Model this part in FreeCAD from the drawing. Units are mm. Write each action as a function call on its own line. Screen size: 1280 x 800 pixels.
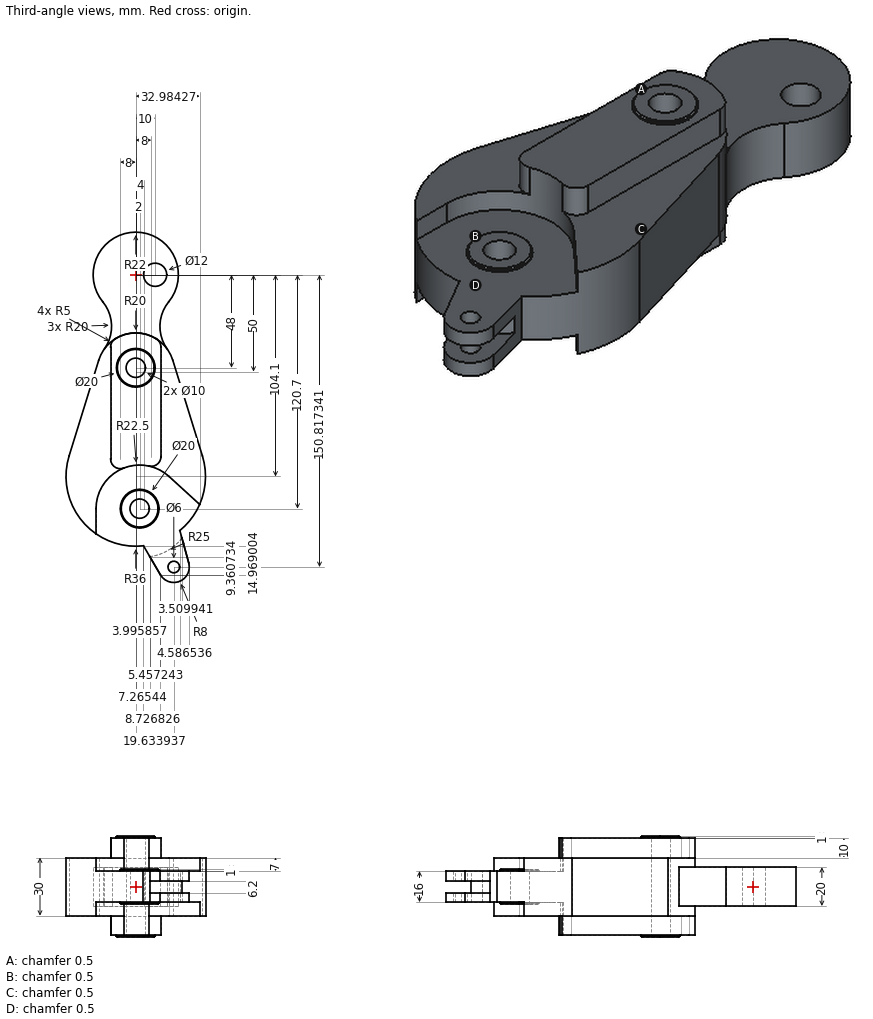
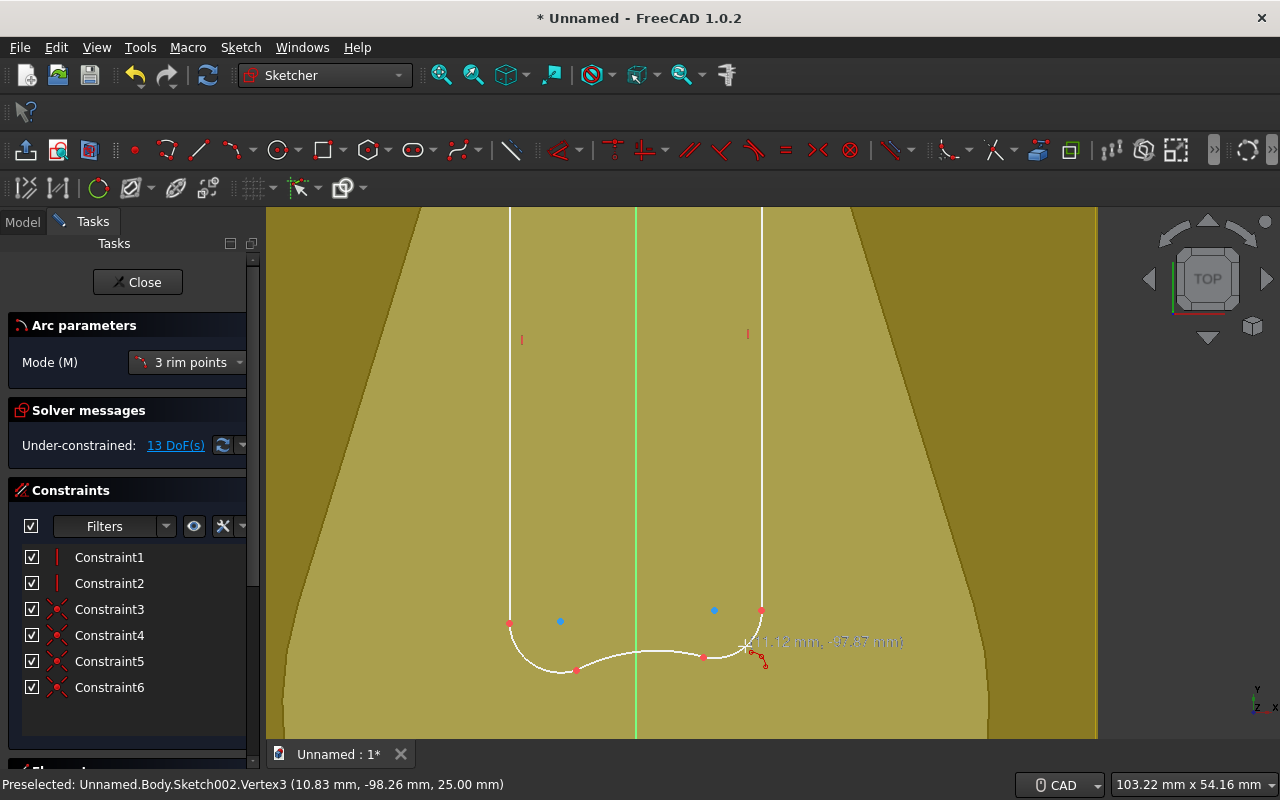
scroll(744, 646, down, 5)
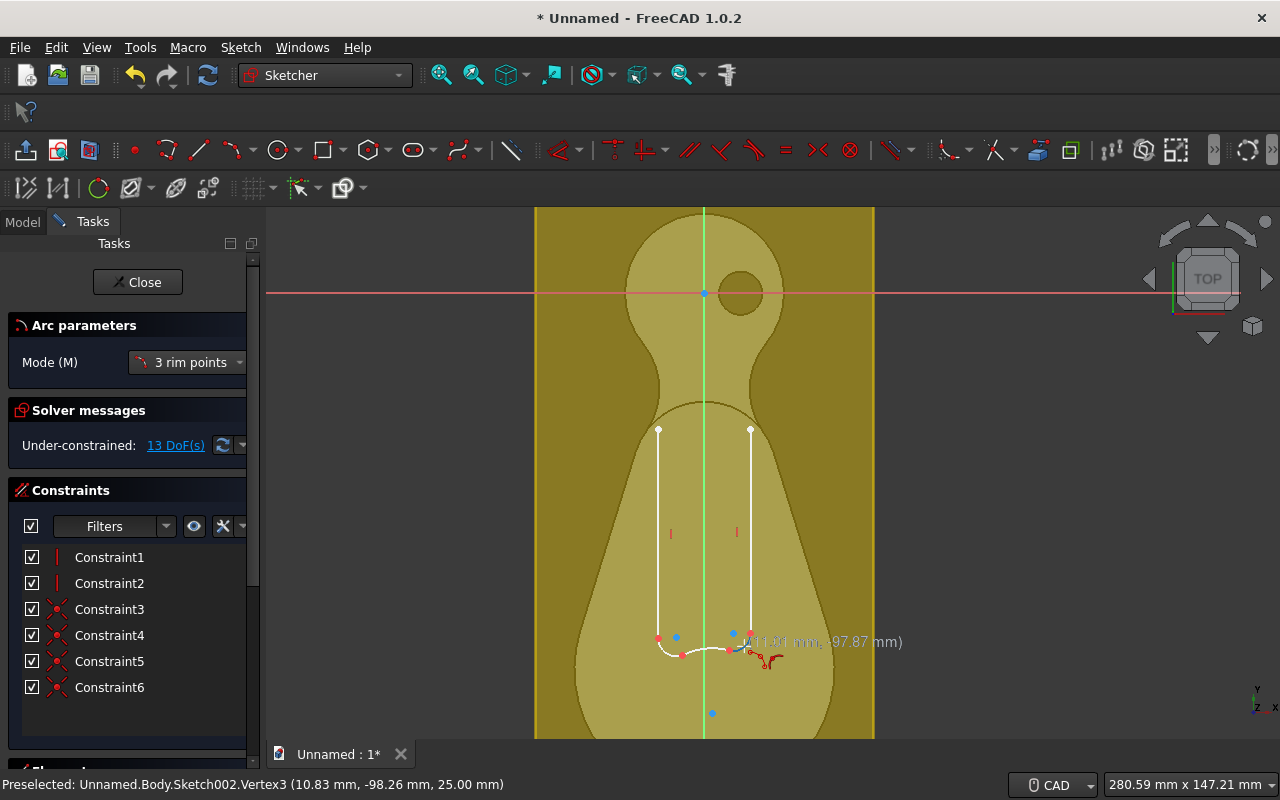
click(751, 430)
click(743, 413)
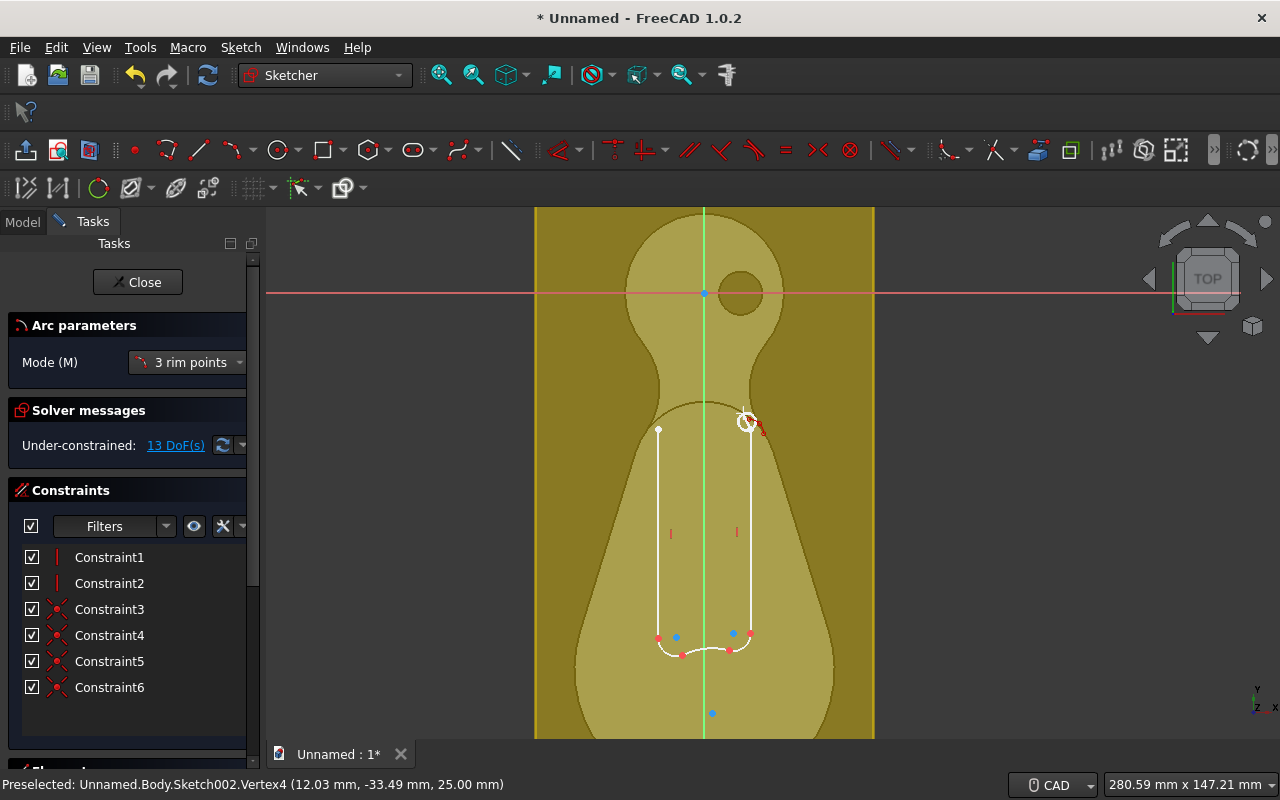
scroll(749, 419, up, 10)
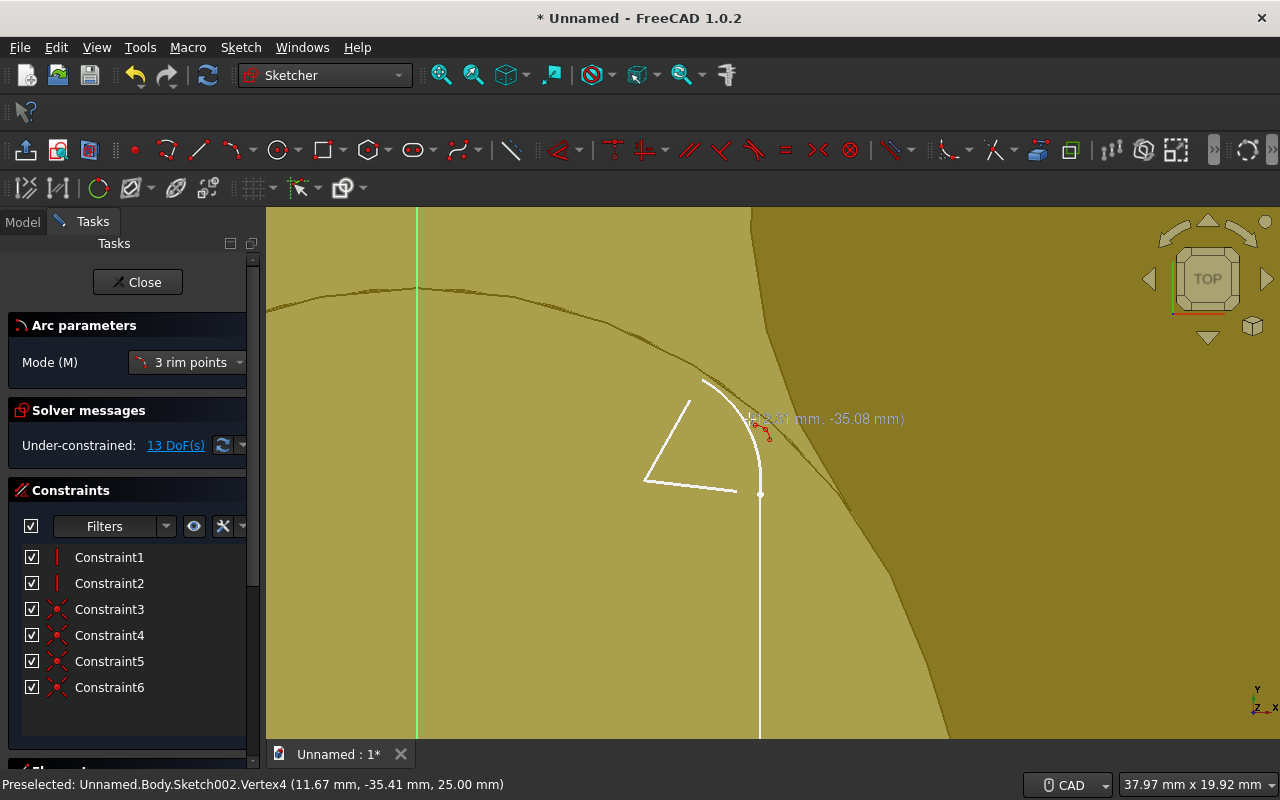
click(748, 419)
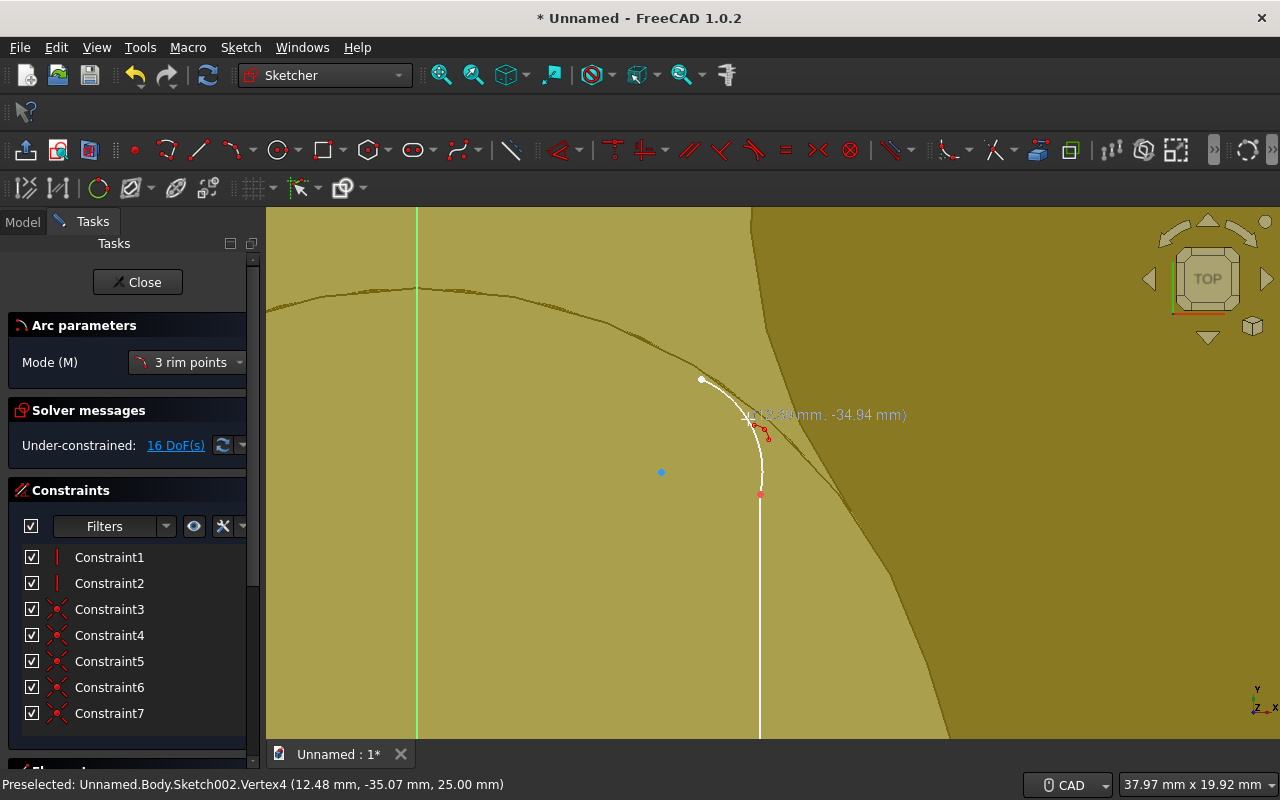
scroll(749, 419, down, 10)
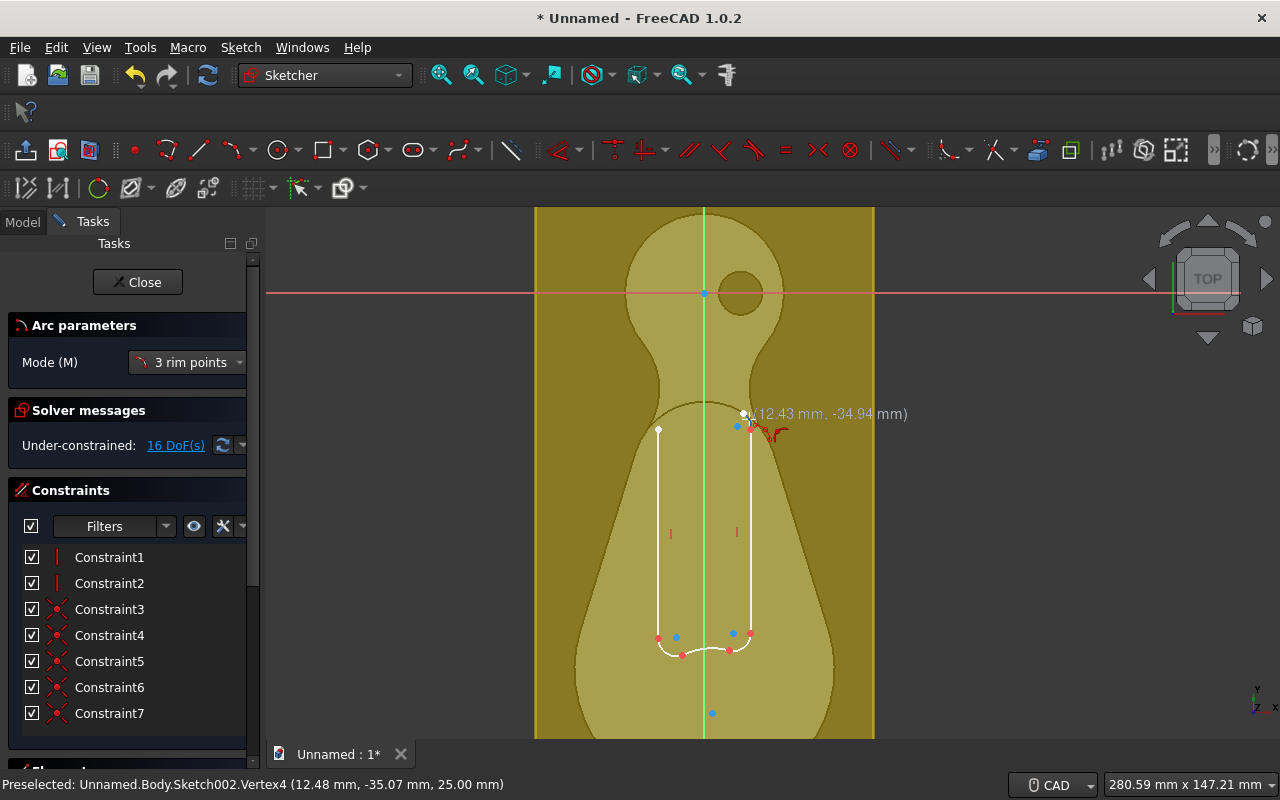
click(743, 414)
click(666, 413)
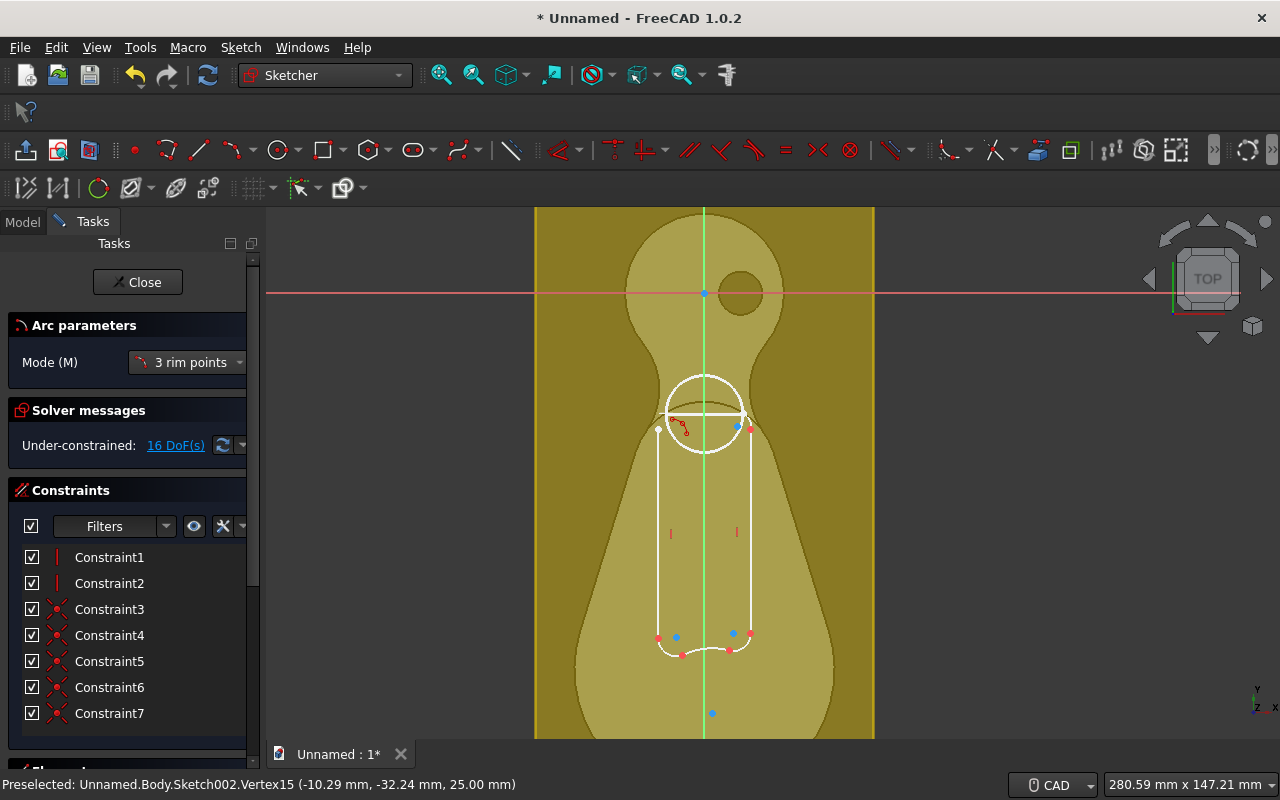
scroll(721, 403, up, 3)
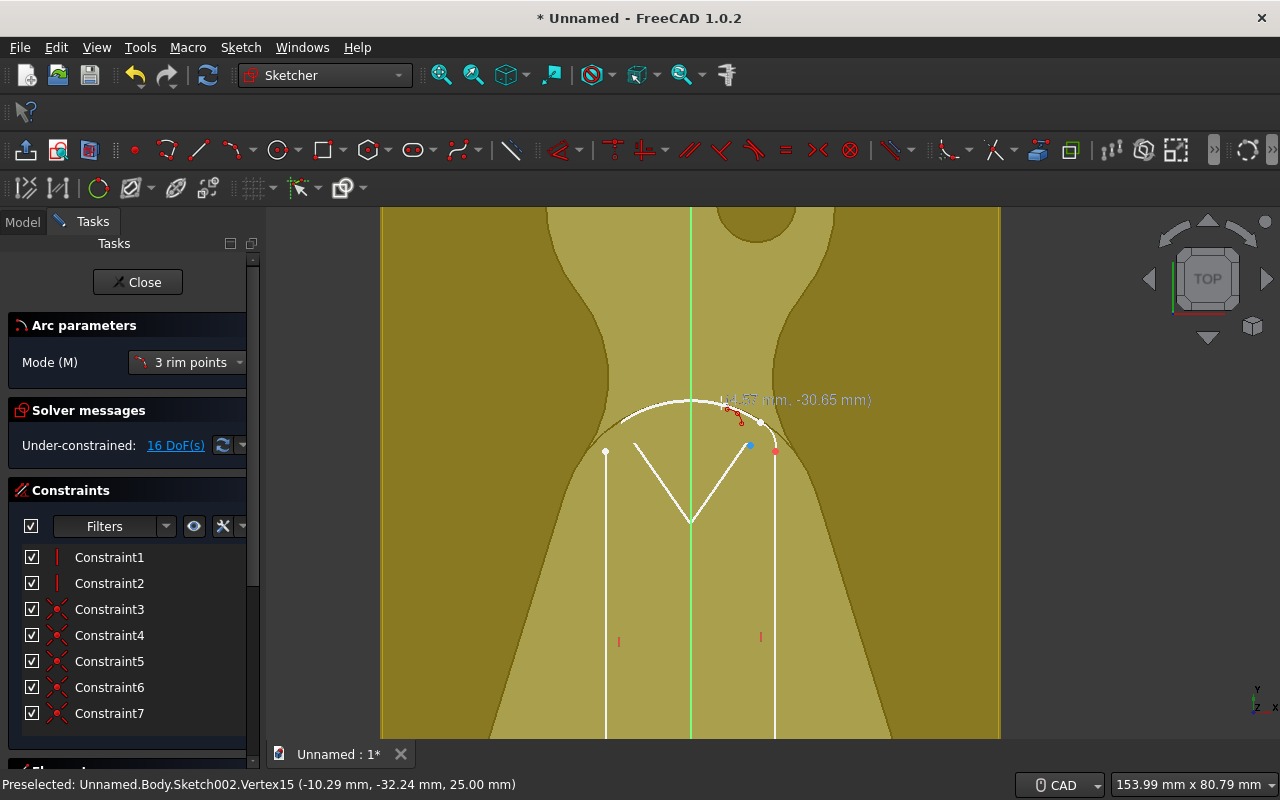
click(720, 404)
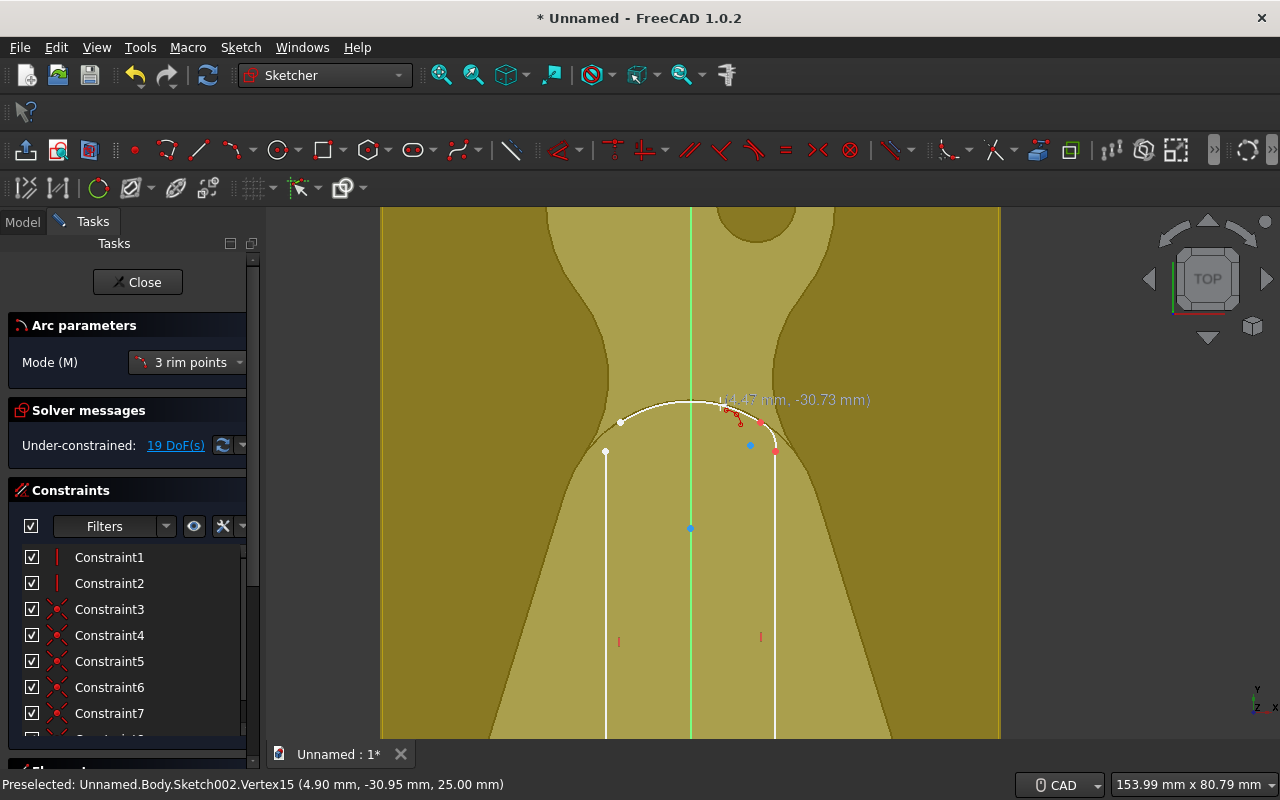
click(620, 423)
click(606, 451)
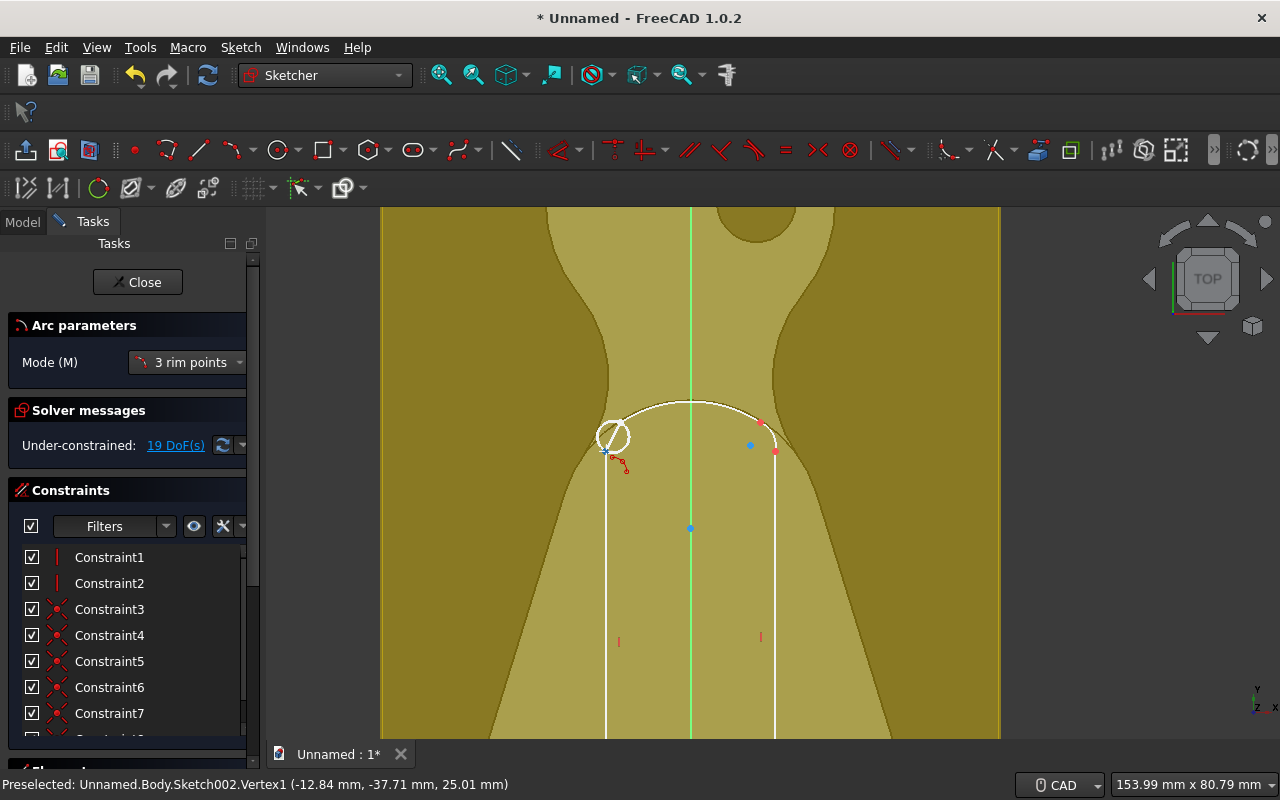
scroll(609, 432, up, 7)